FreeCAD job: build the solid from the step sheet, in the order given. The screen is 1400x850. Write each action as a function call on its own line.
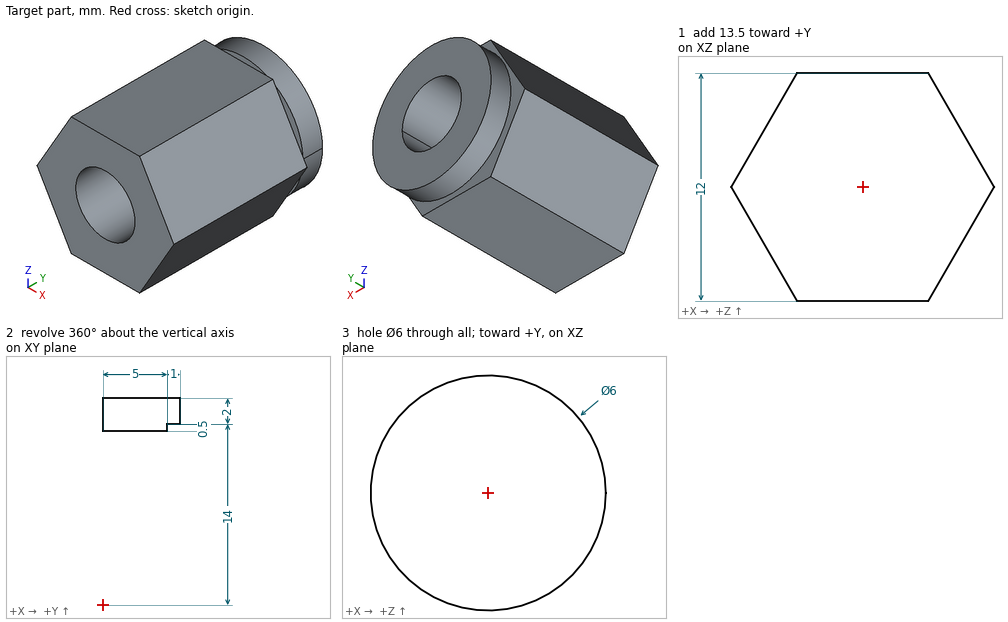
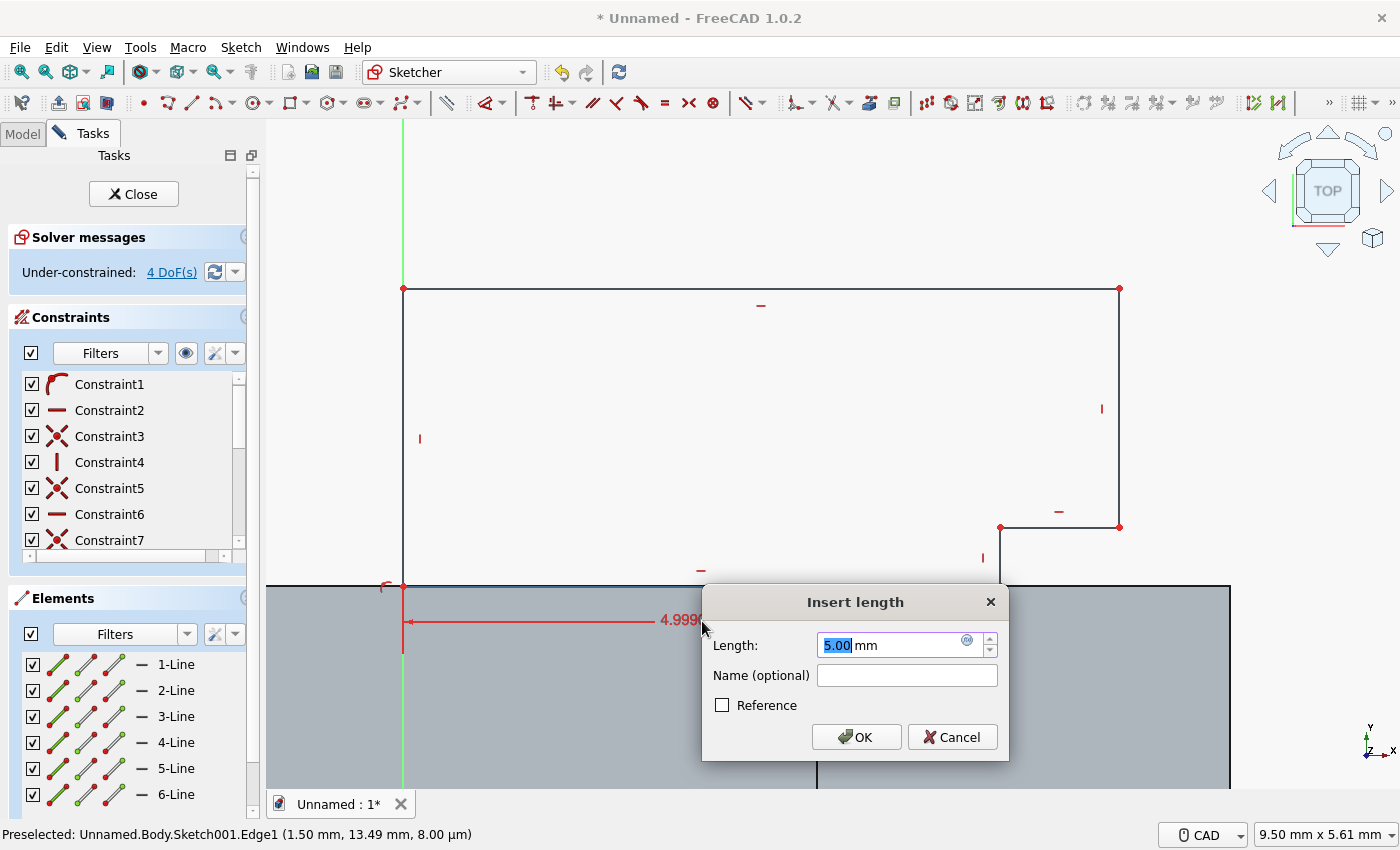
text(5)
key(Return)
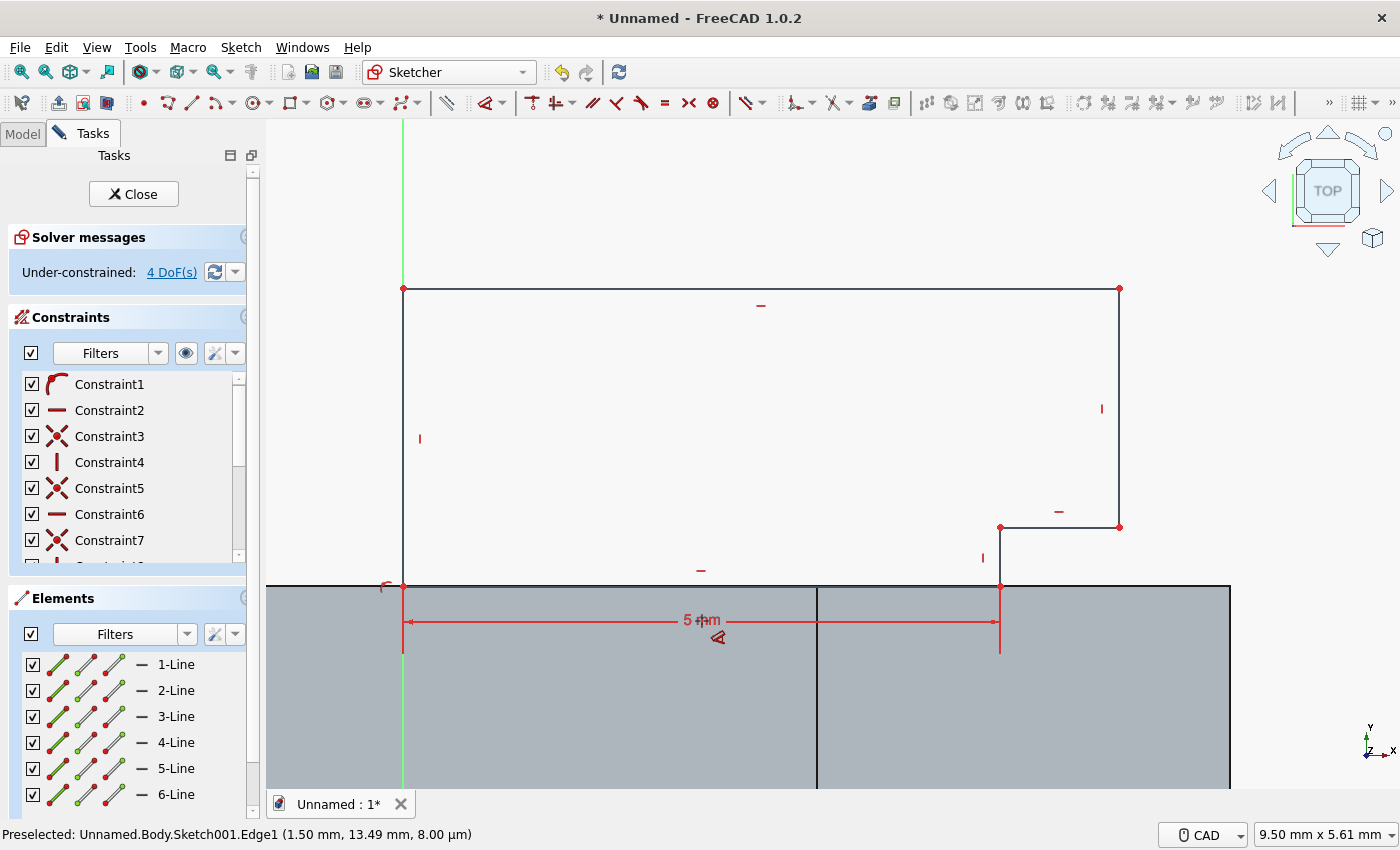
click(1036, 528)
click(1060, 562)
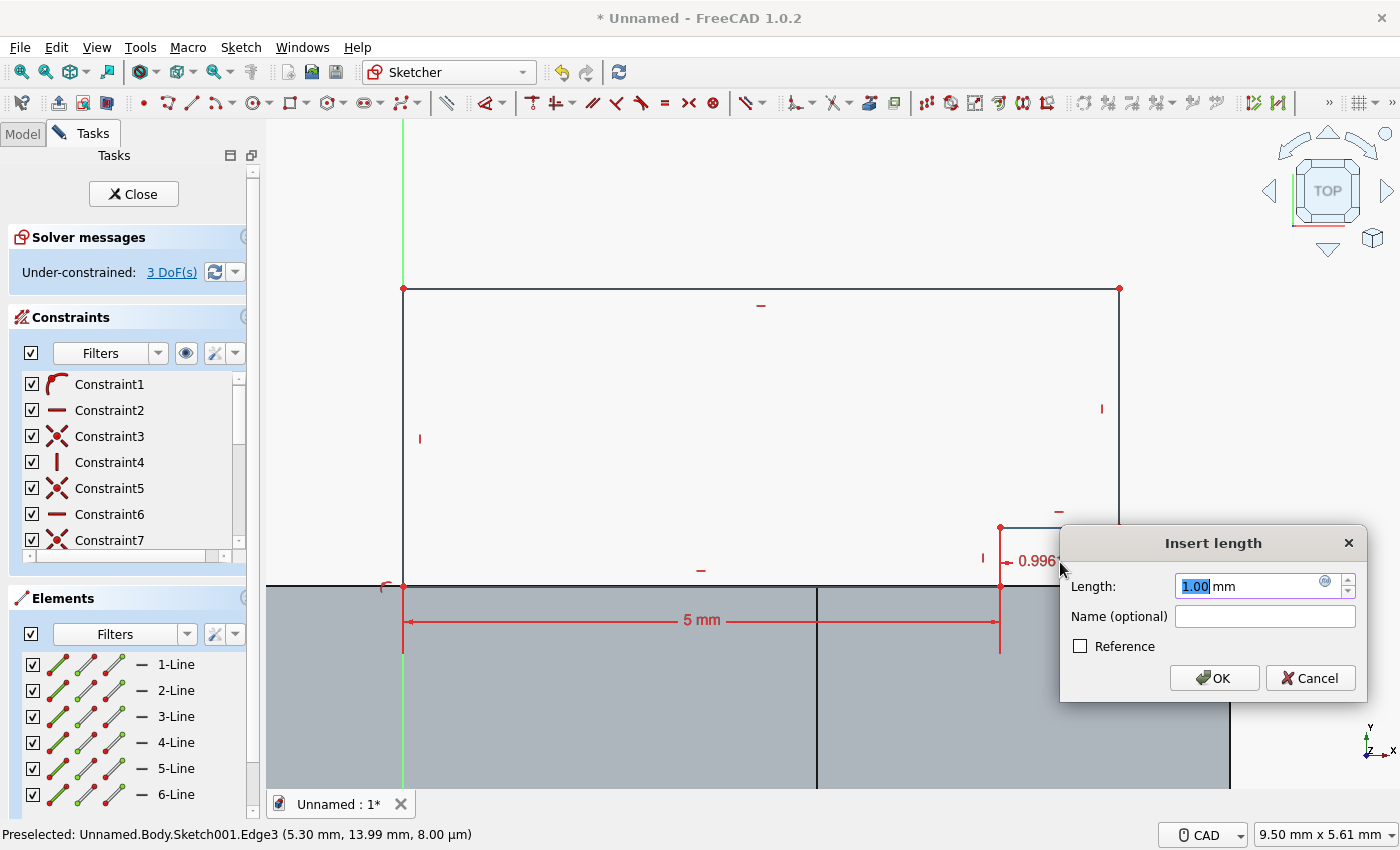
text(1)
key(Return)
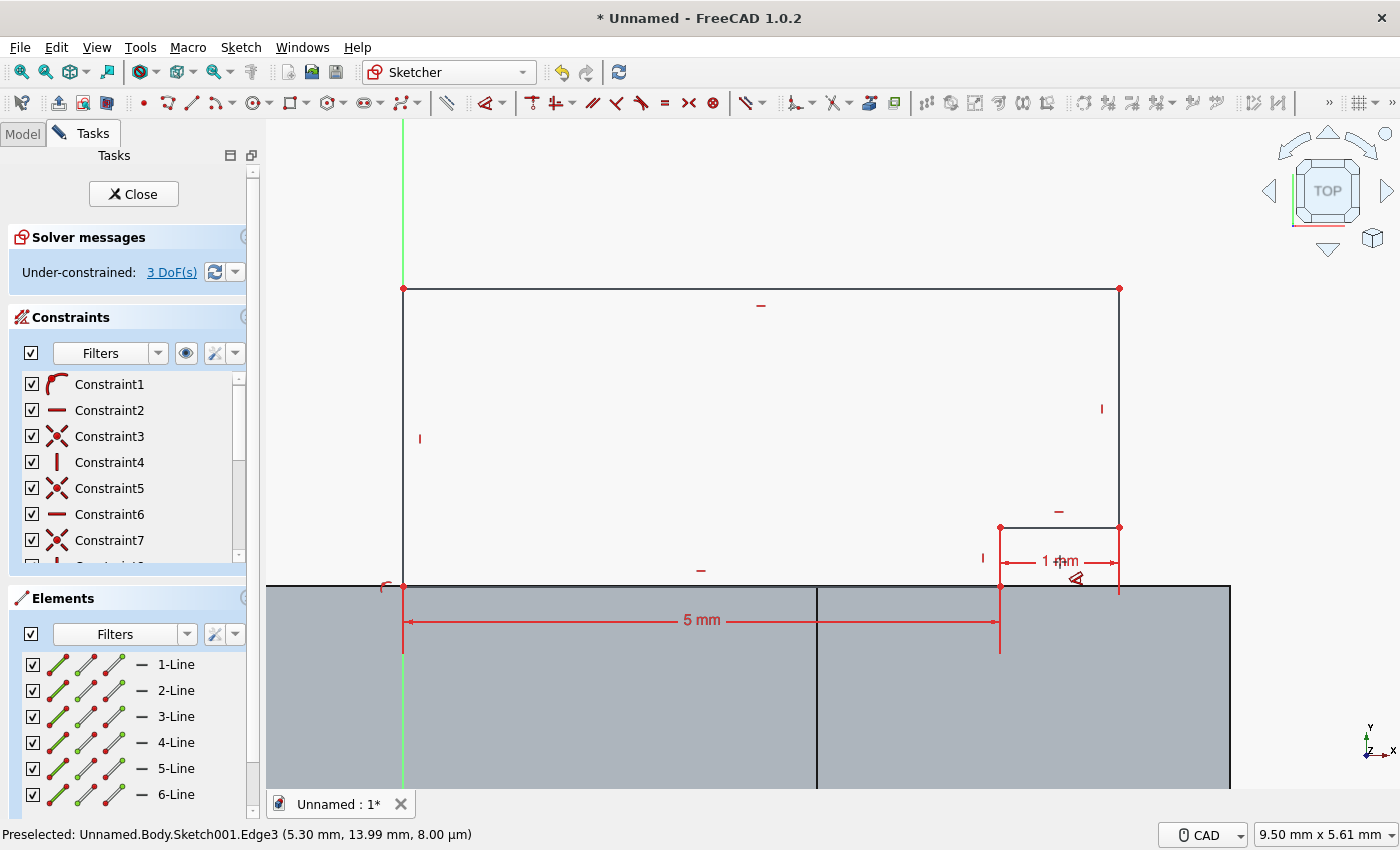
click(1119, 456)
click(1153, 408)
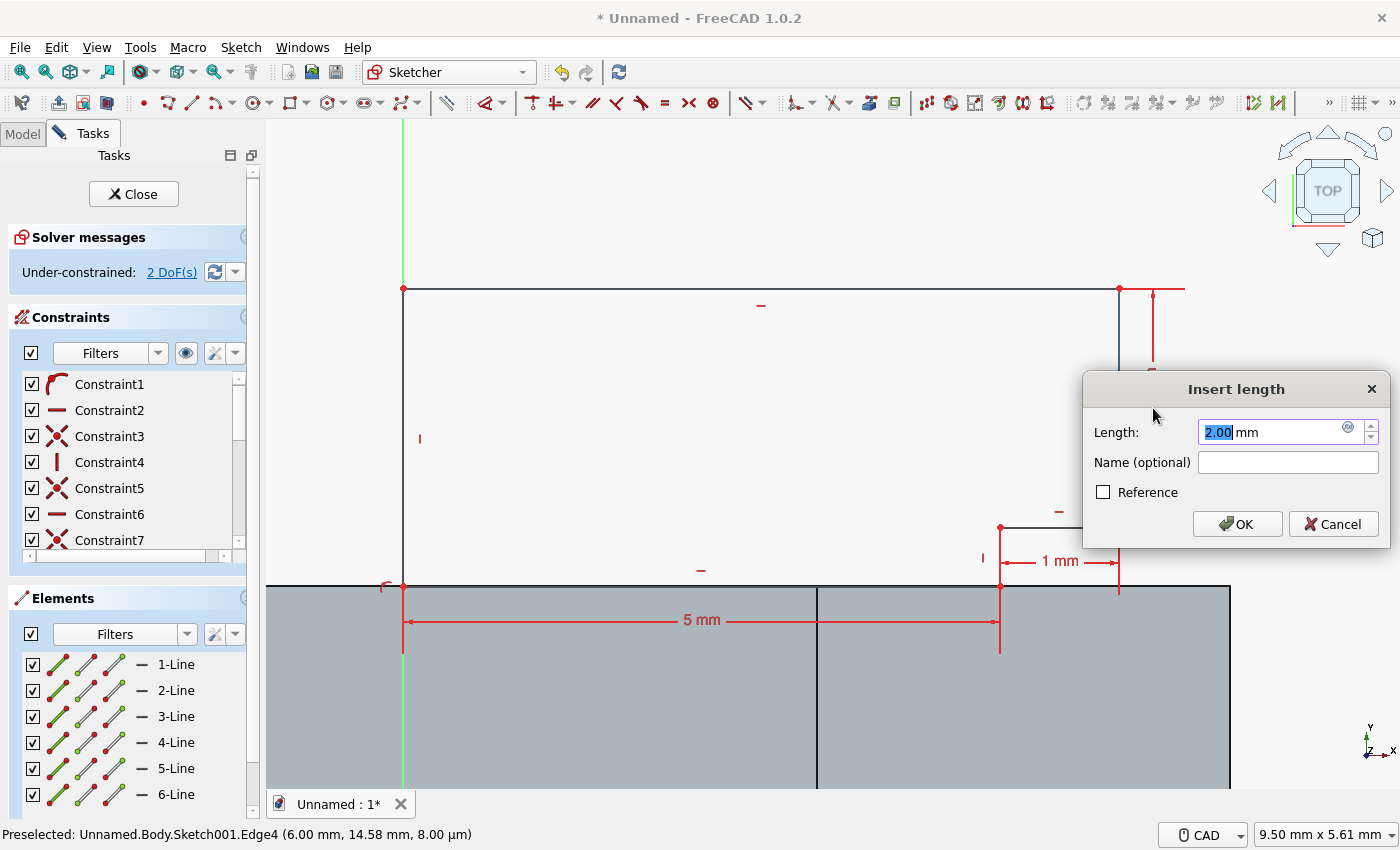
text(2)
key(Return)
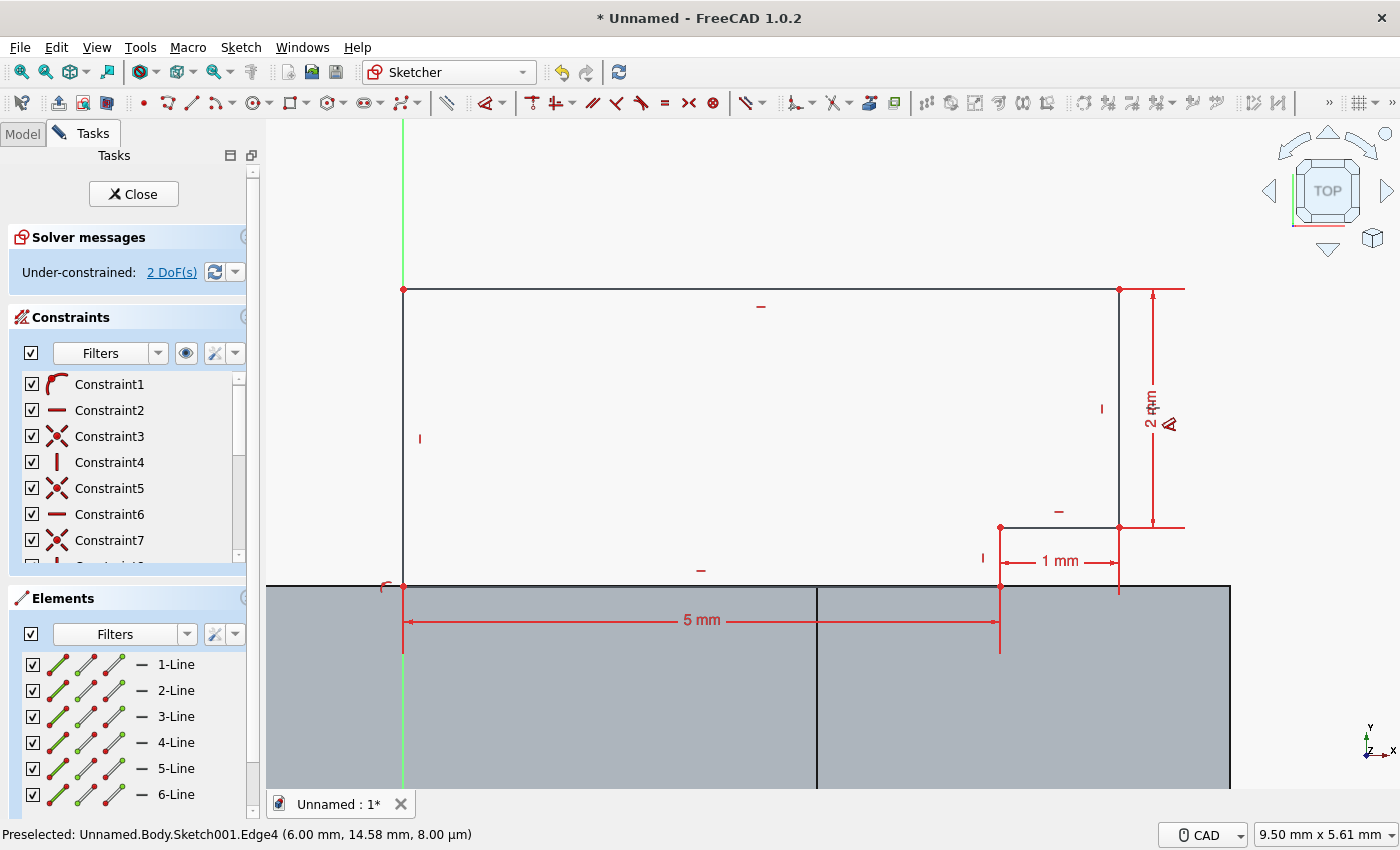
click(1000, 569)
click(966, 557)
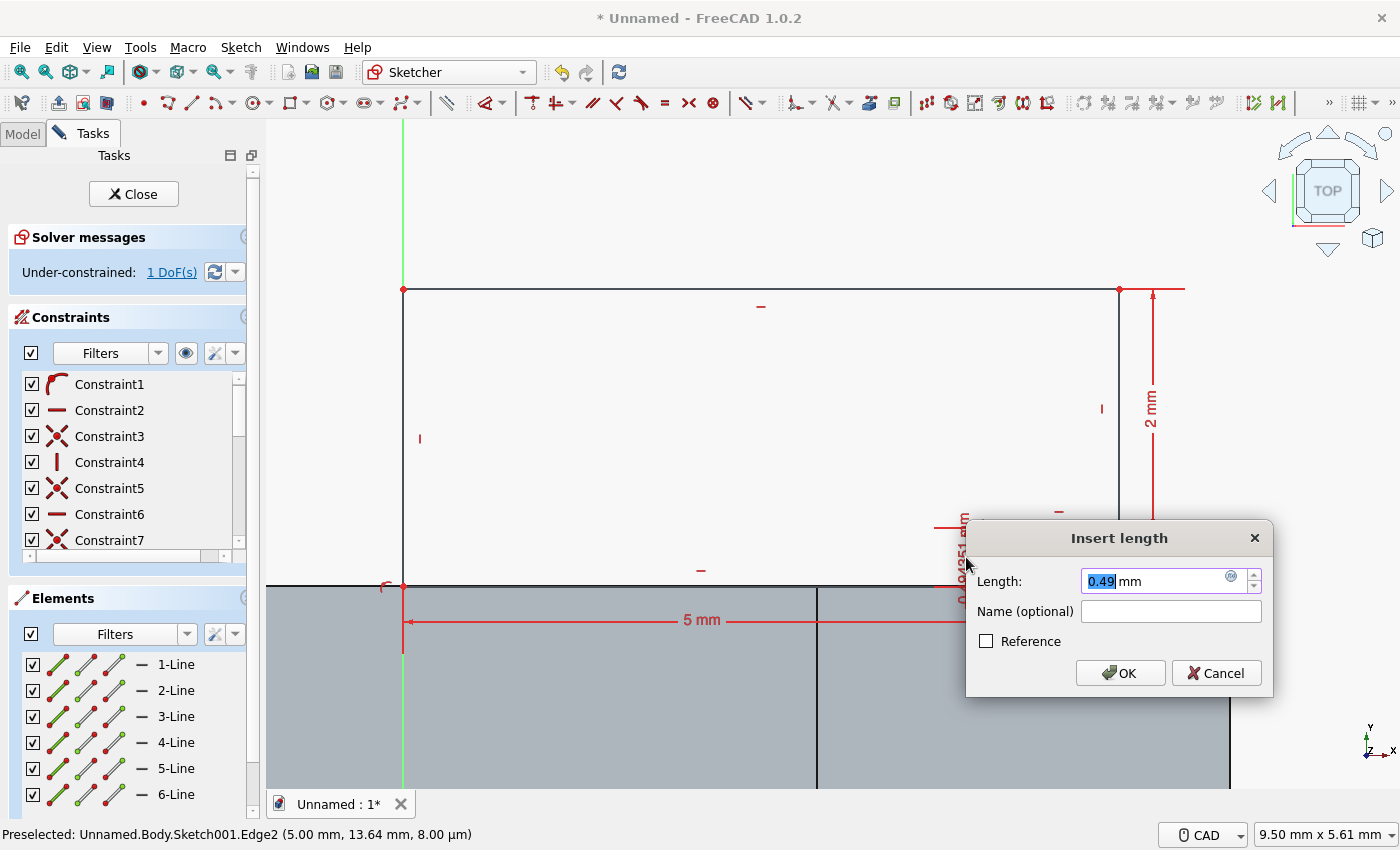
text(0.5)
key(Return)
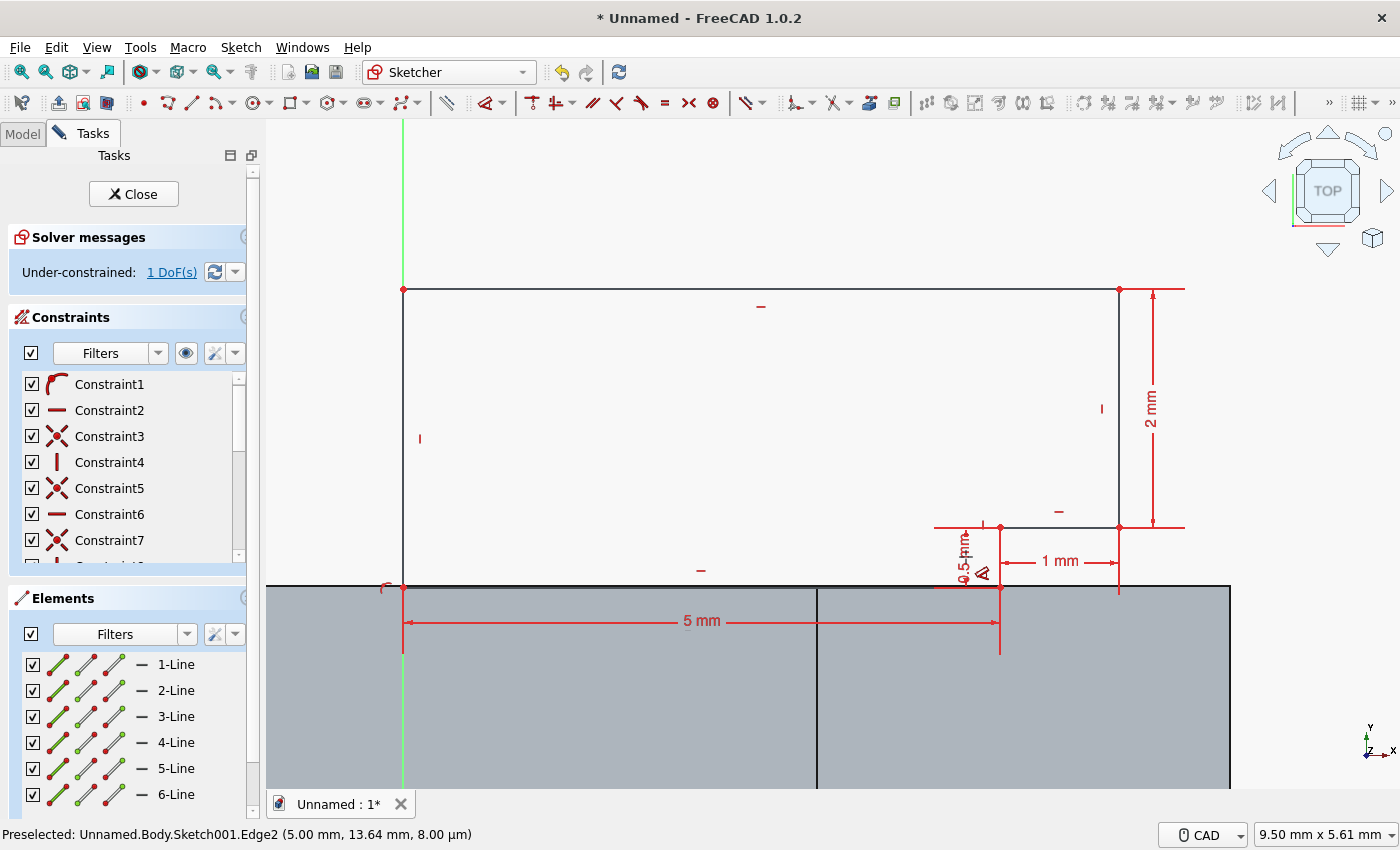
click(1000, 528)
click(369, 644)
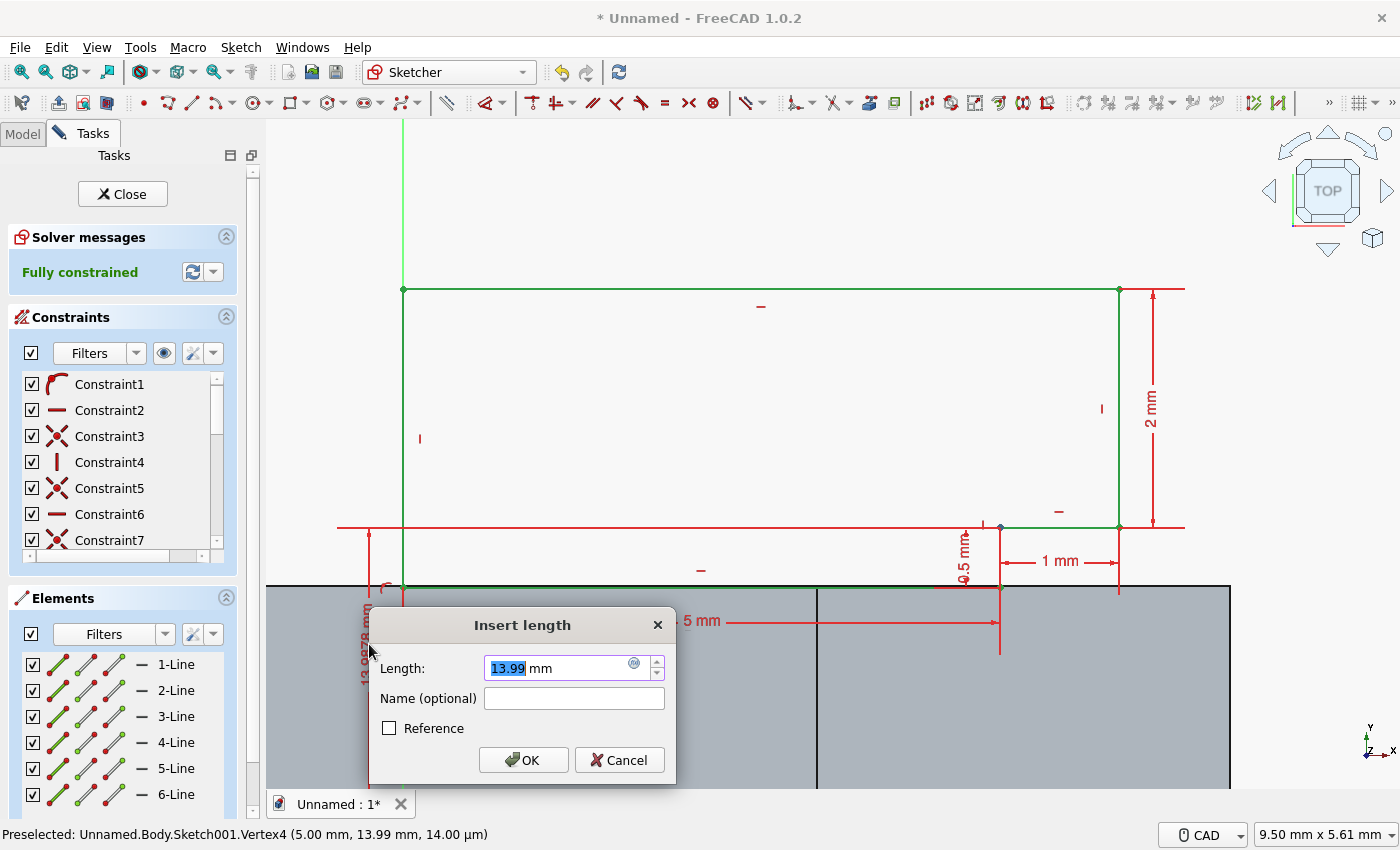
text(14)
key(Return)
key(Escape)